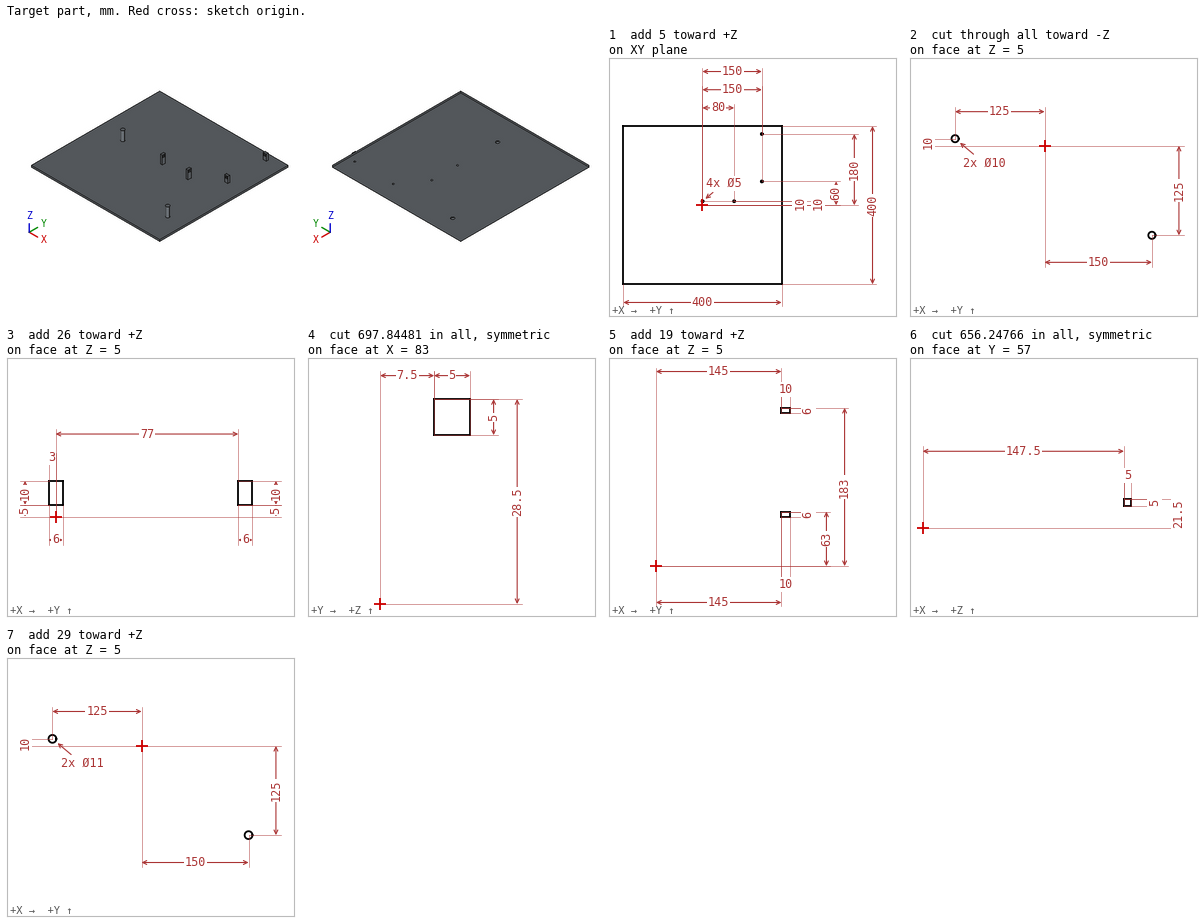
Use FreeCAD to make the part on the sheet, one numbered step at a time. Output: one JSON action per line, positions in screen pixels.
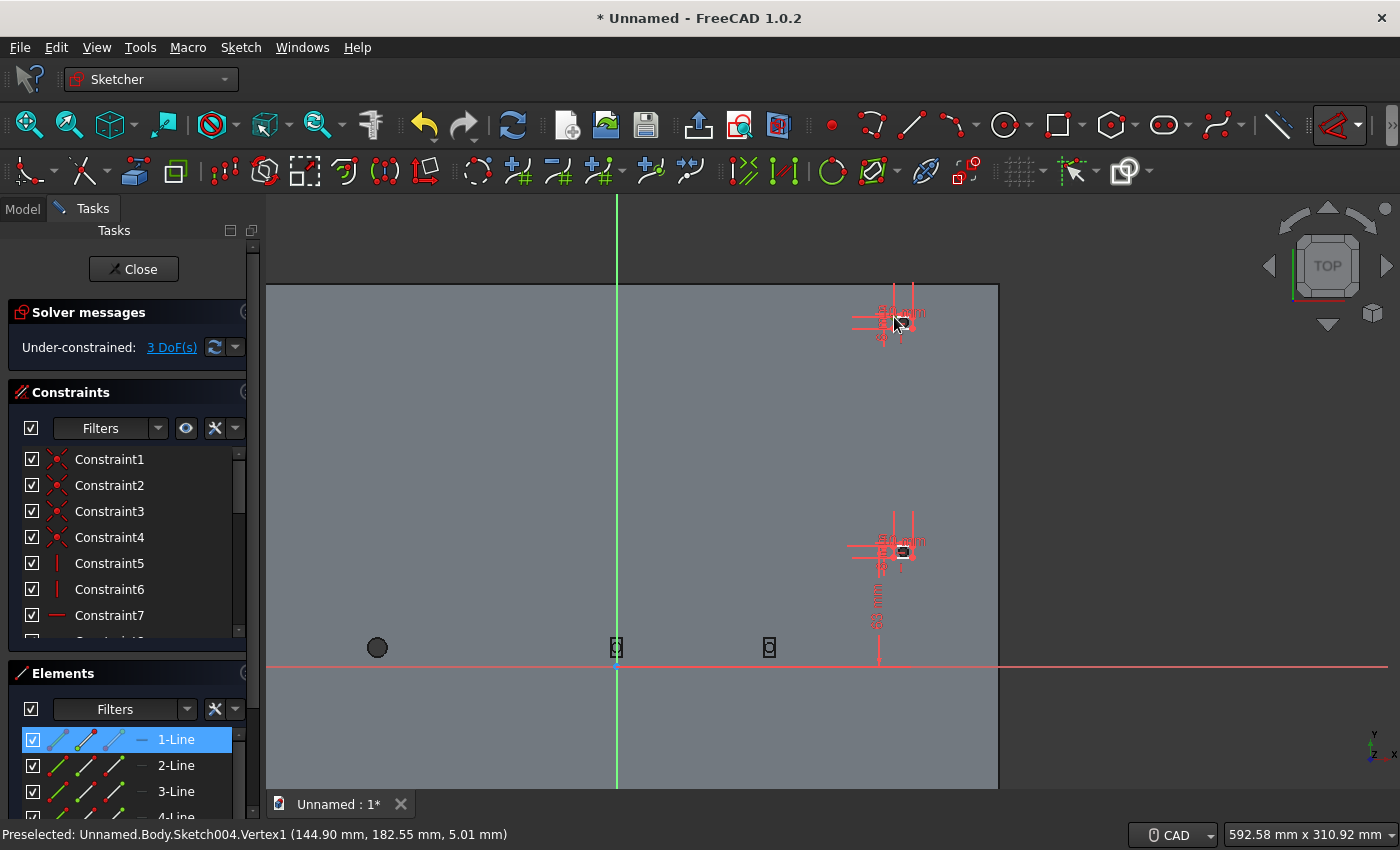
{"action": "key", "text": "l"}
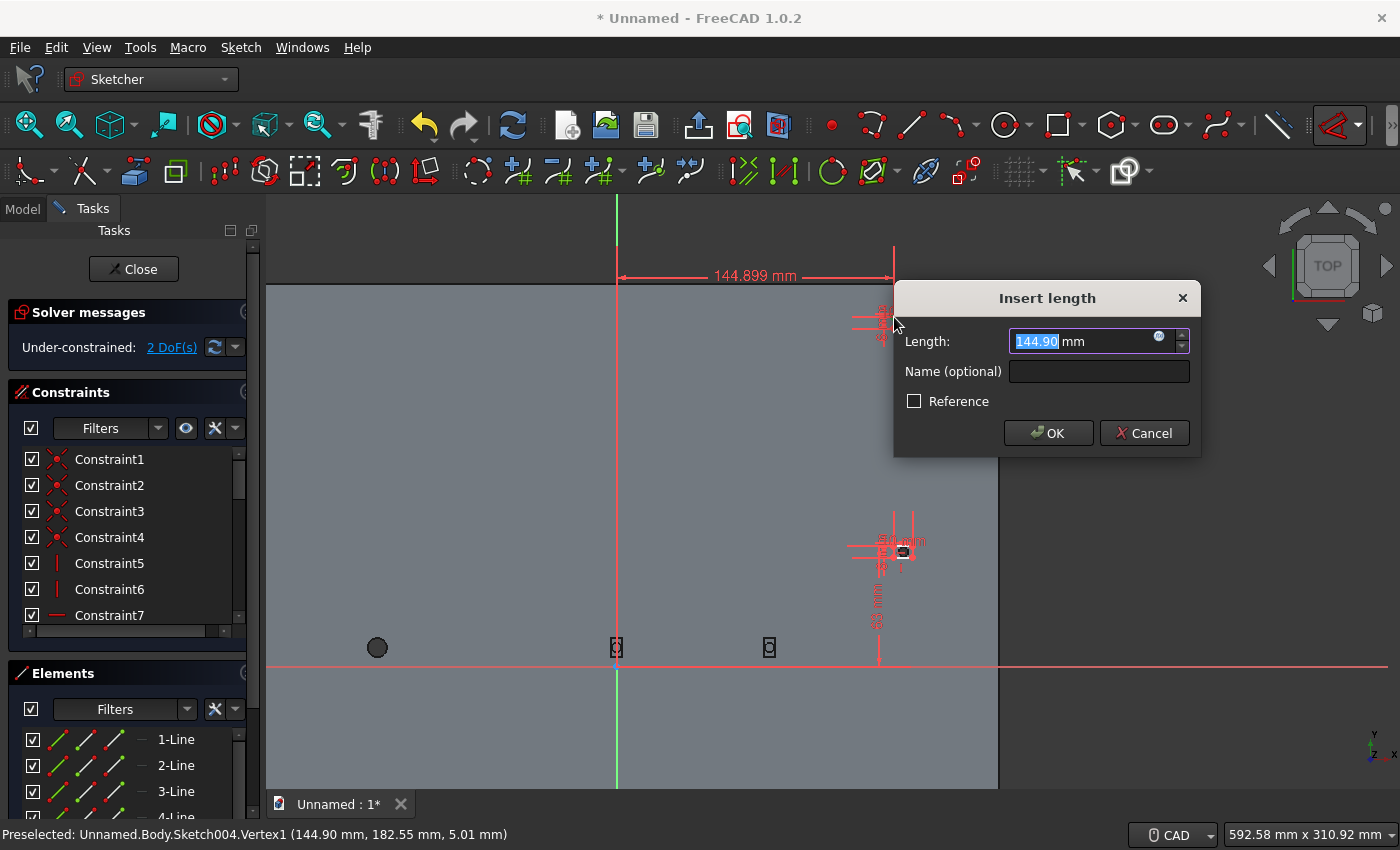
{"action": "type", "text": "145"}
{"action": "key", "text": "Return"}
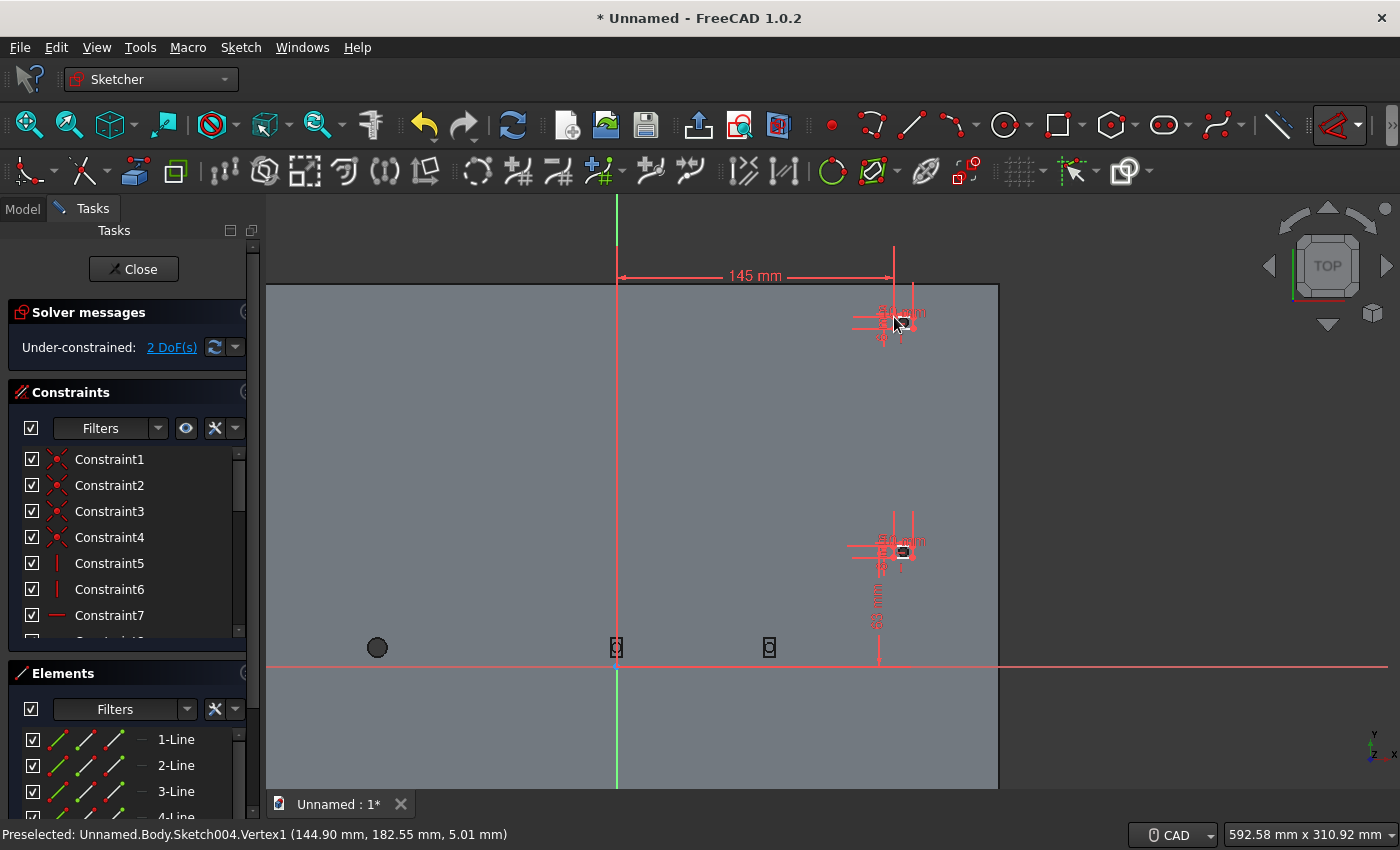
{"action": "left_click", "coordinate": [894, 317]}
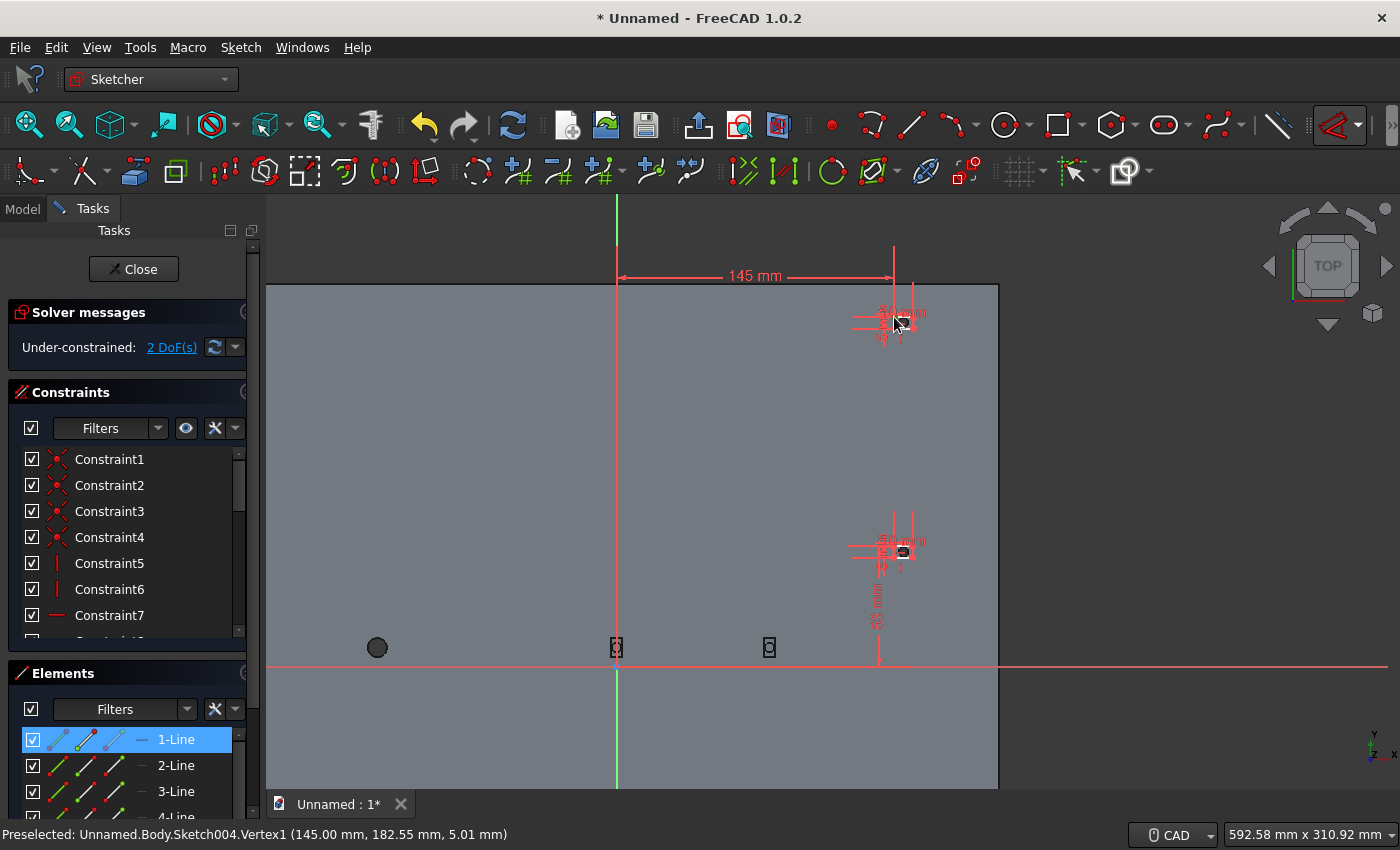
{"action": "key", "text": "i"}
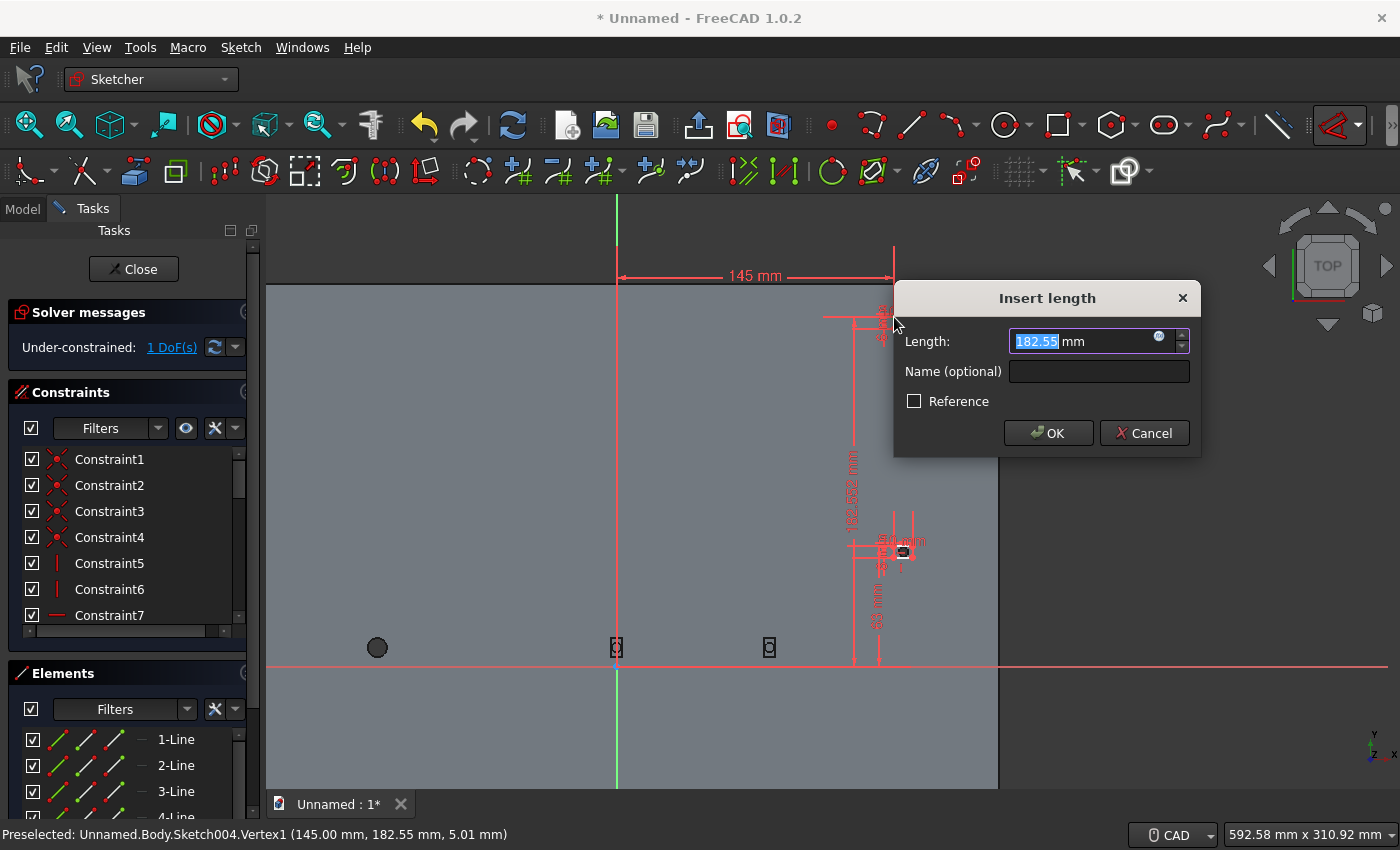
{"action": "type", "text": "183"}
{"action": "key", "text": "Return"}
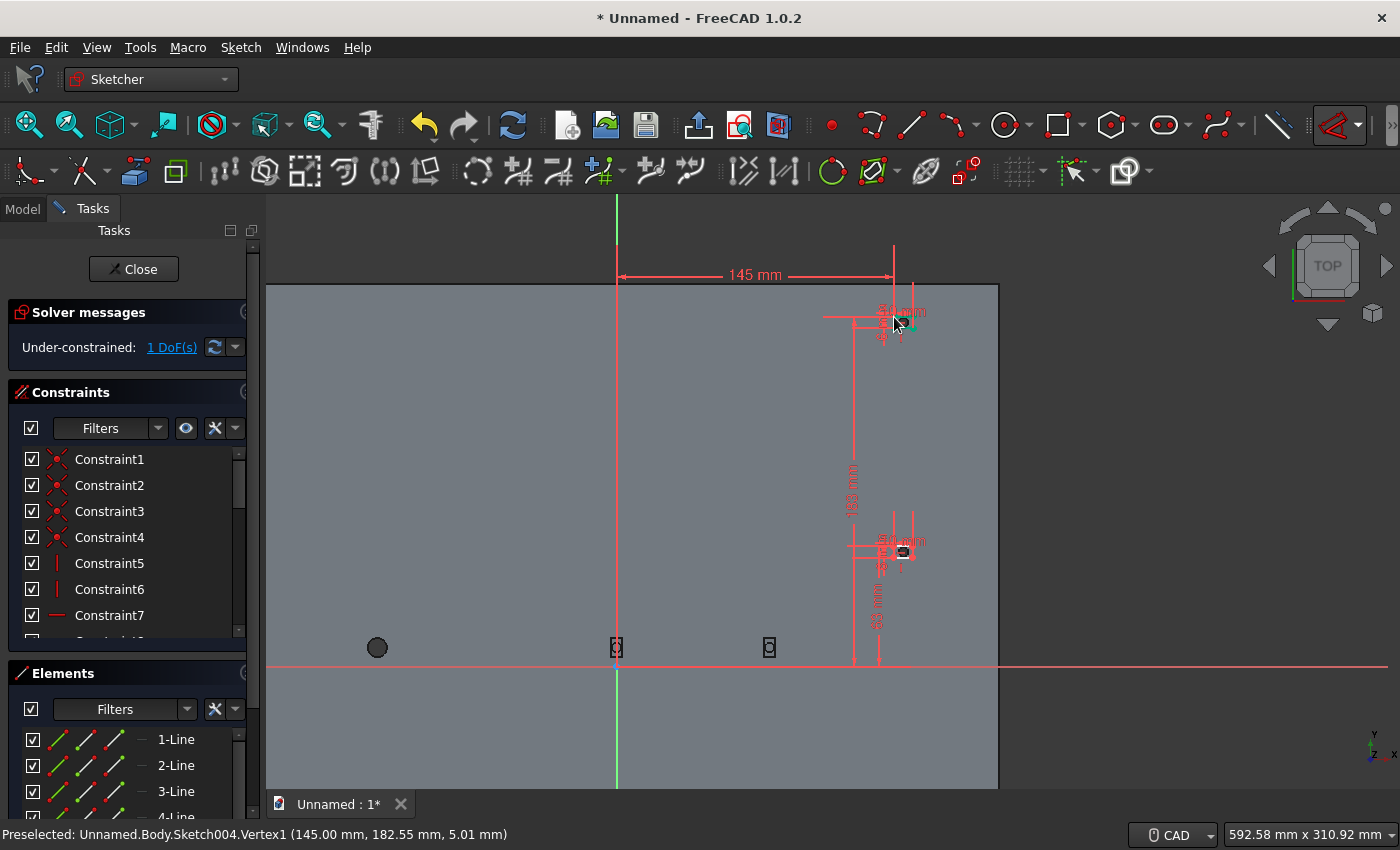
{"action": "left_click", "coordinate": [894, 546]}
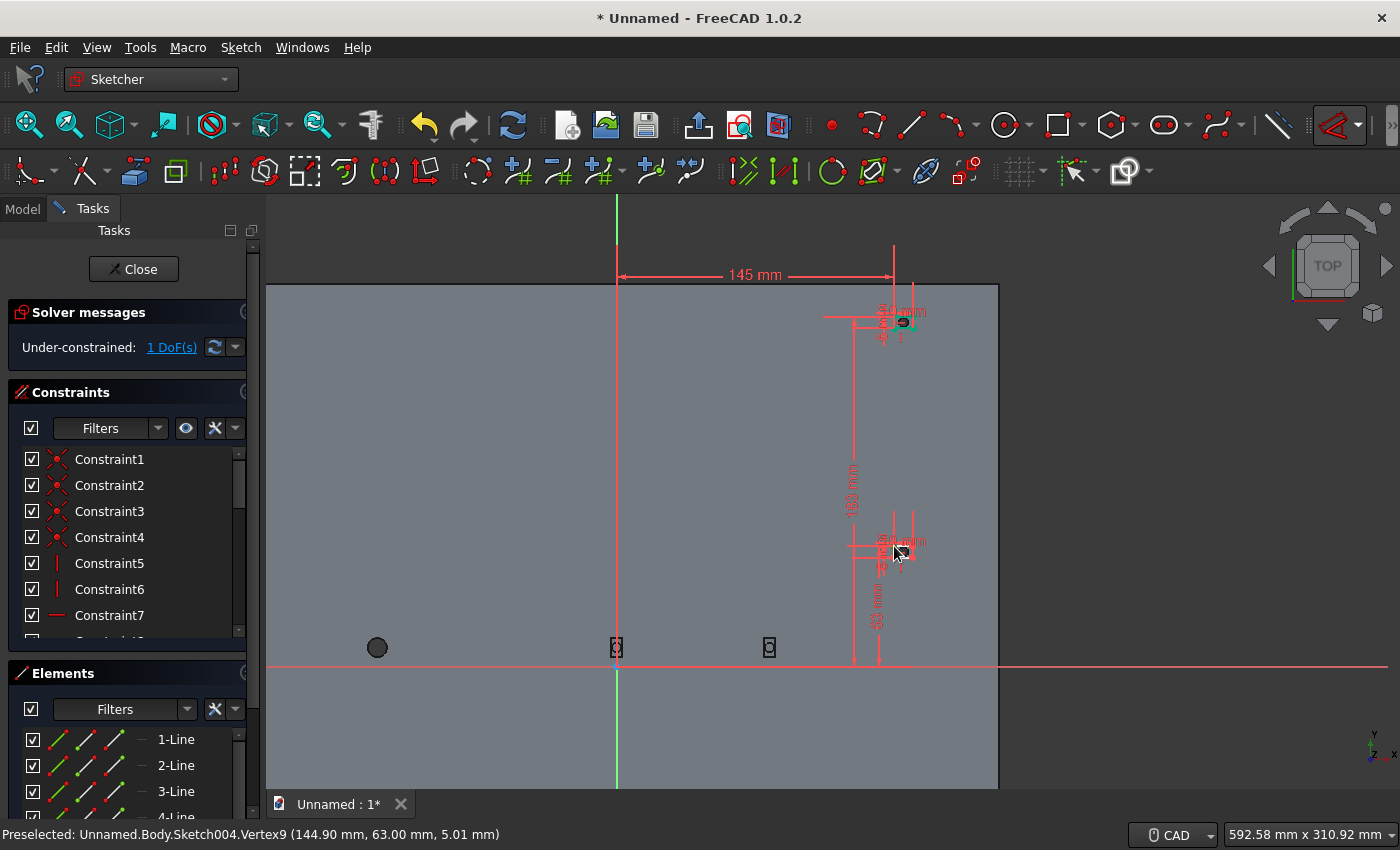
{"action": "left_click", "coordinate": [1360, 126]}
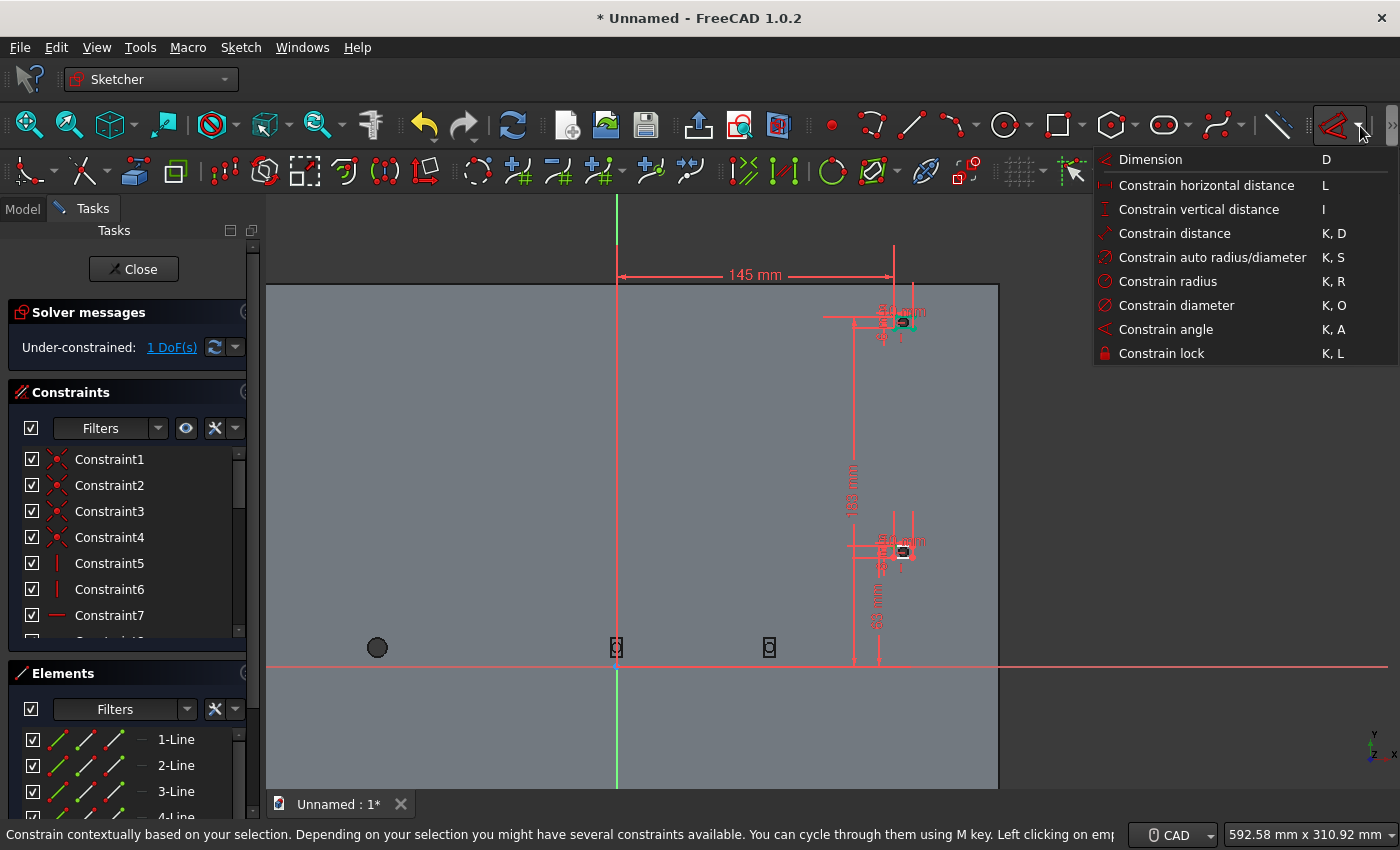
{"action": "left_click", "coordinate": [1246, 185]}